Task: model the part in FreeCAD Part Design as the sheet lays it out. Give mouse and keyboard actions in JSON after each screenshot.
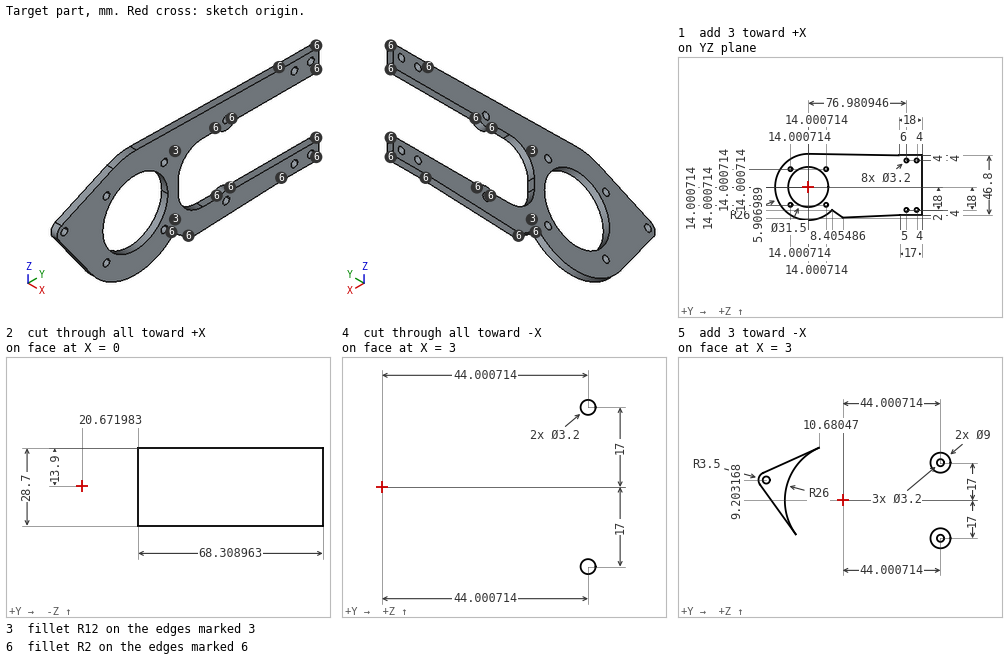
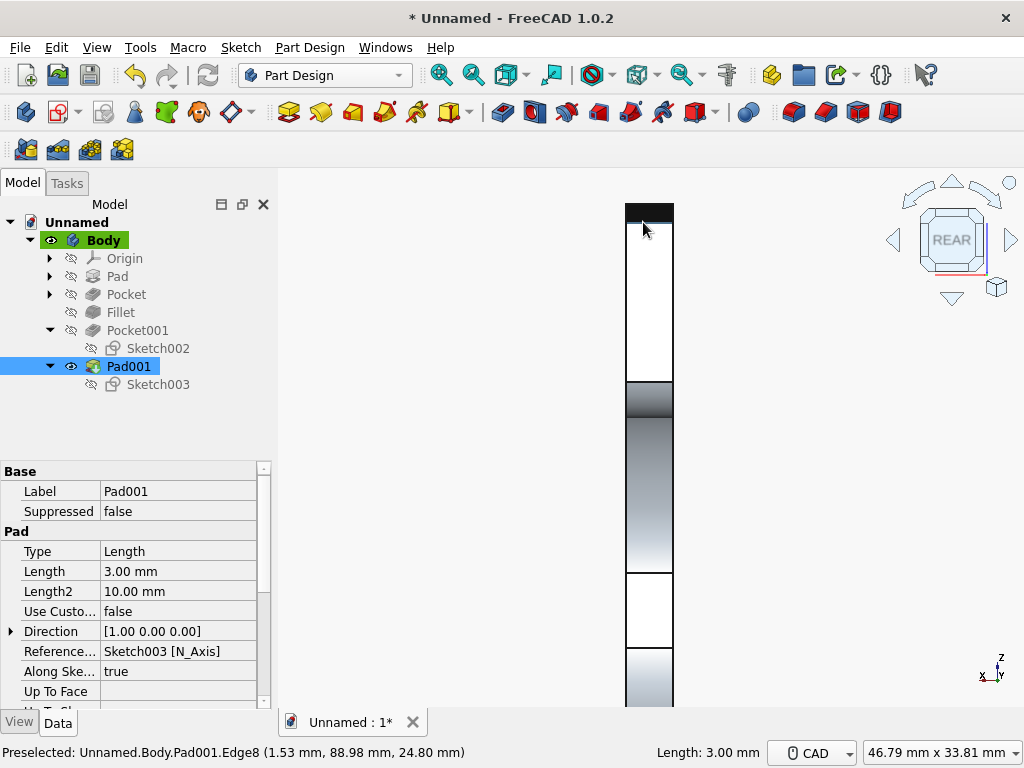
{"action": "left_click", "coordinate": [649, 381], "text": "ctrl"}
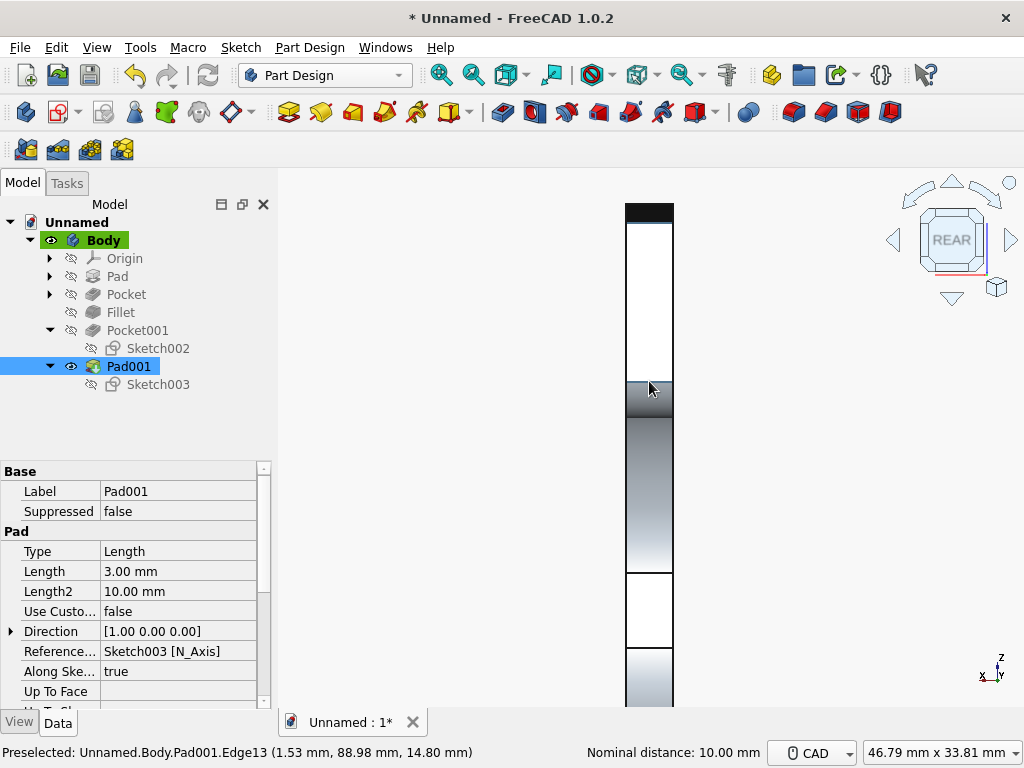
{"action": "left_click", "coordinate": [442, 76]}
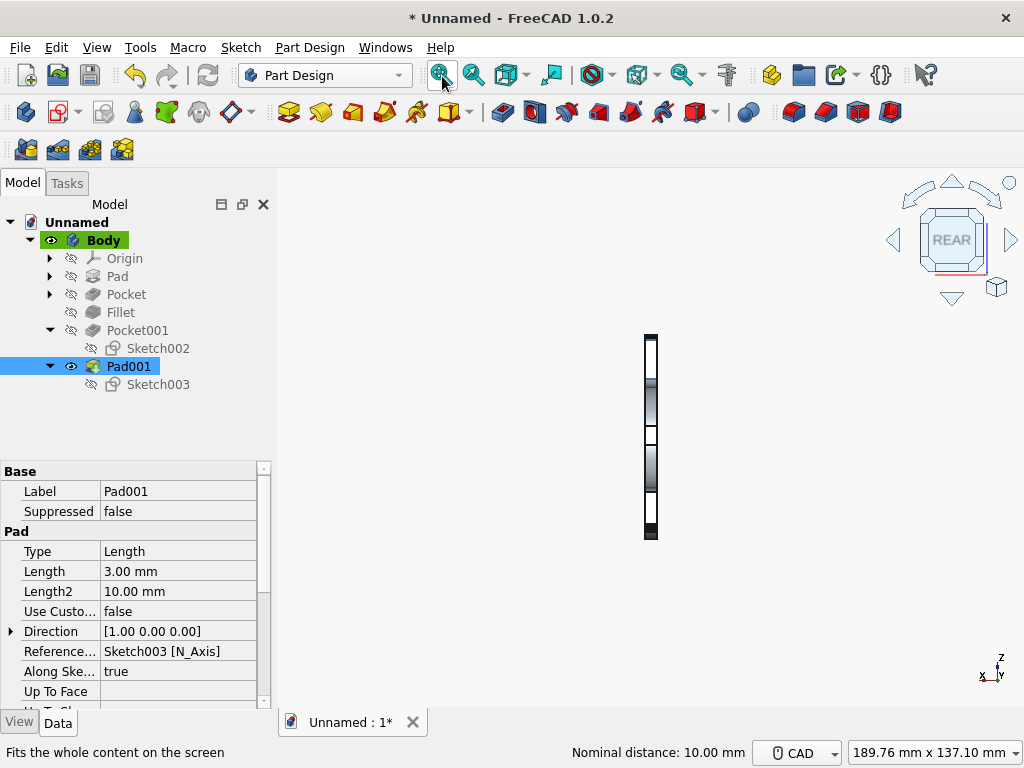
{"action": "key", "text": "6"}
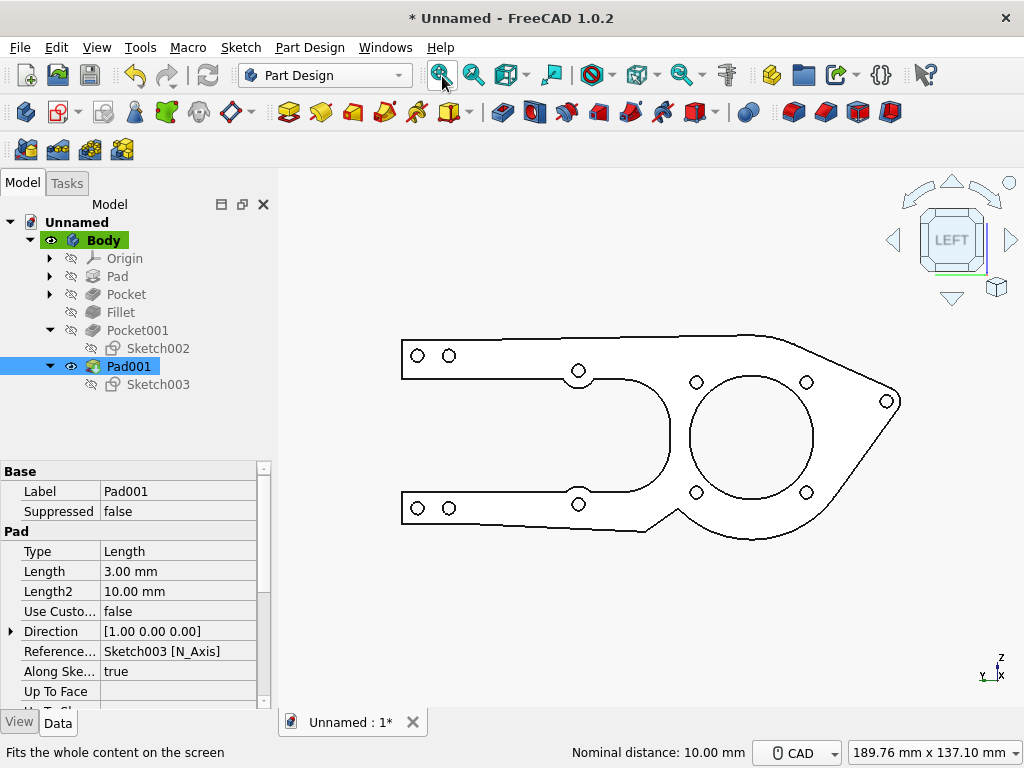
{"action": "scroll", "coordinate": [563, 378], "scroll_direction": "up", "scroll_amount": 7}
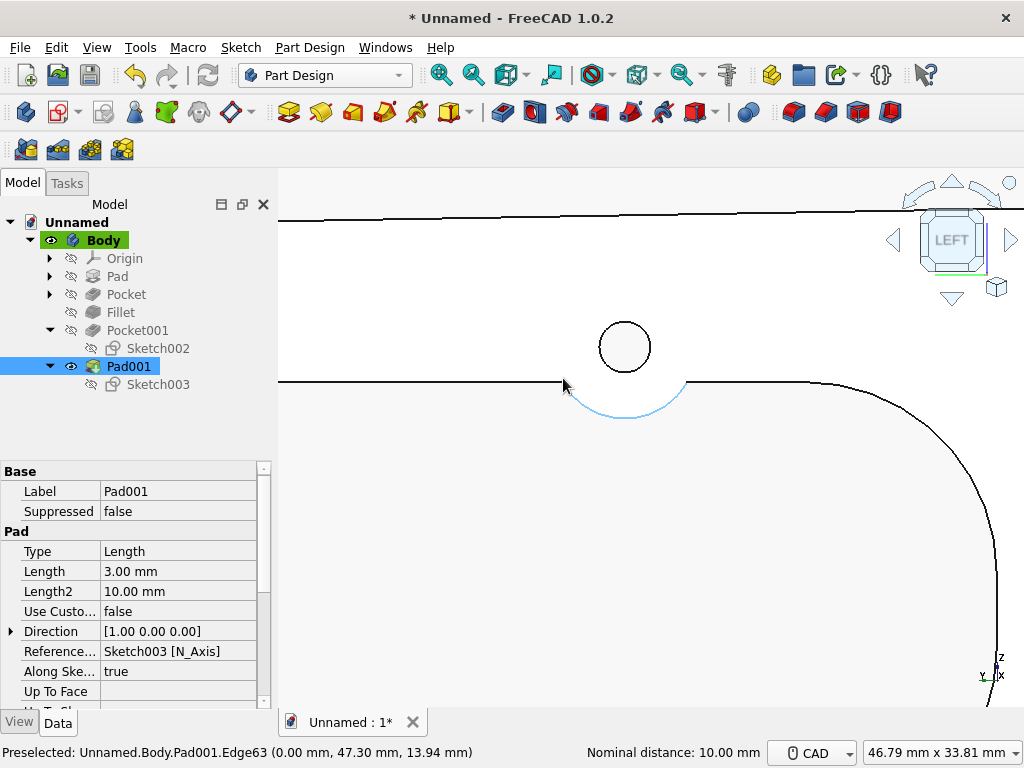
{"action": "left_click", "coordinate": [442, 76]}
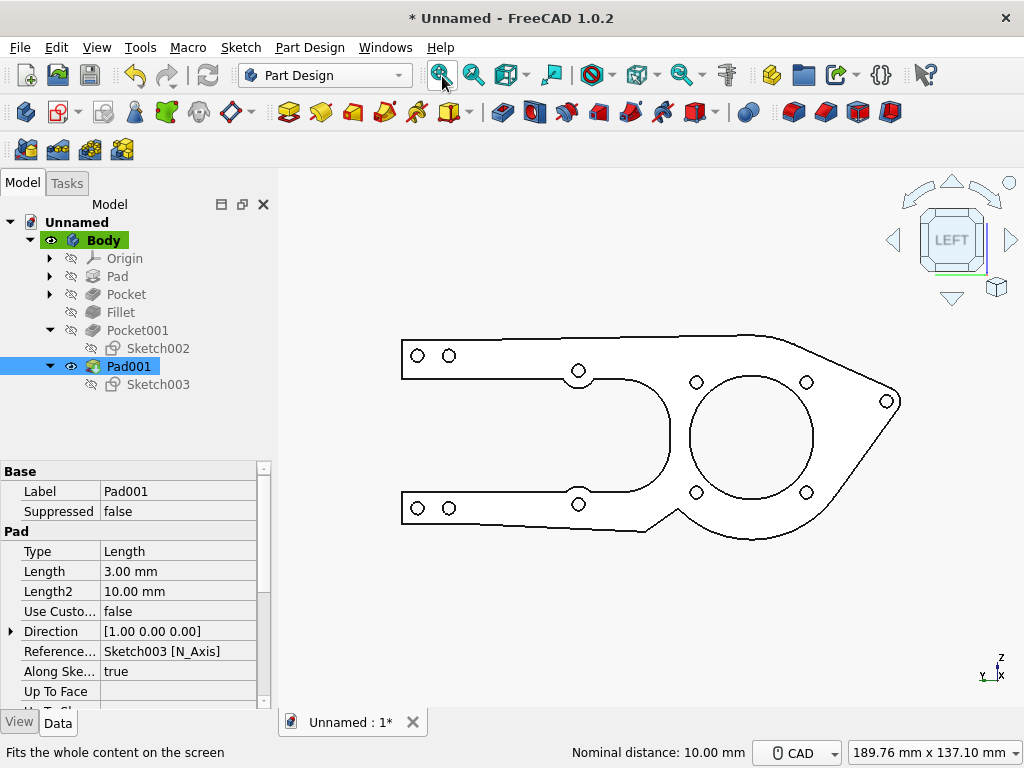
{"action": "key", "text": "v 3"}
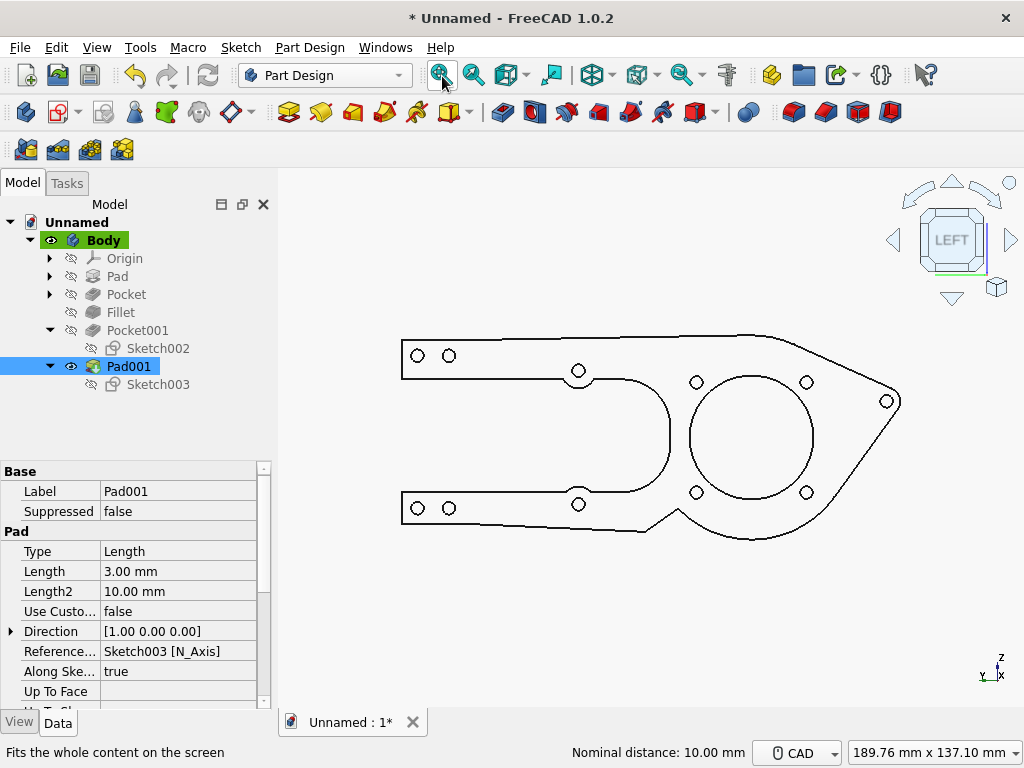
{"action": "key", "text": "0"}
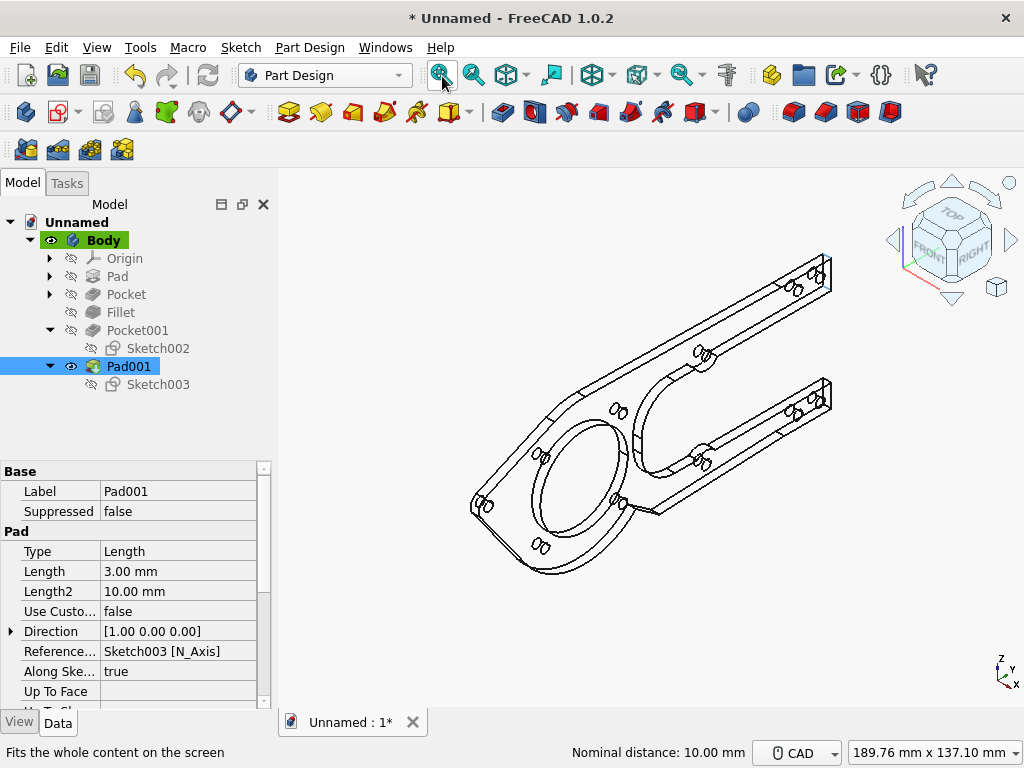
{"action": "left_click", "coordinate": [689, 364], "text": "ctrl"}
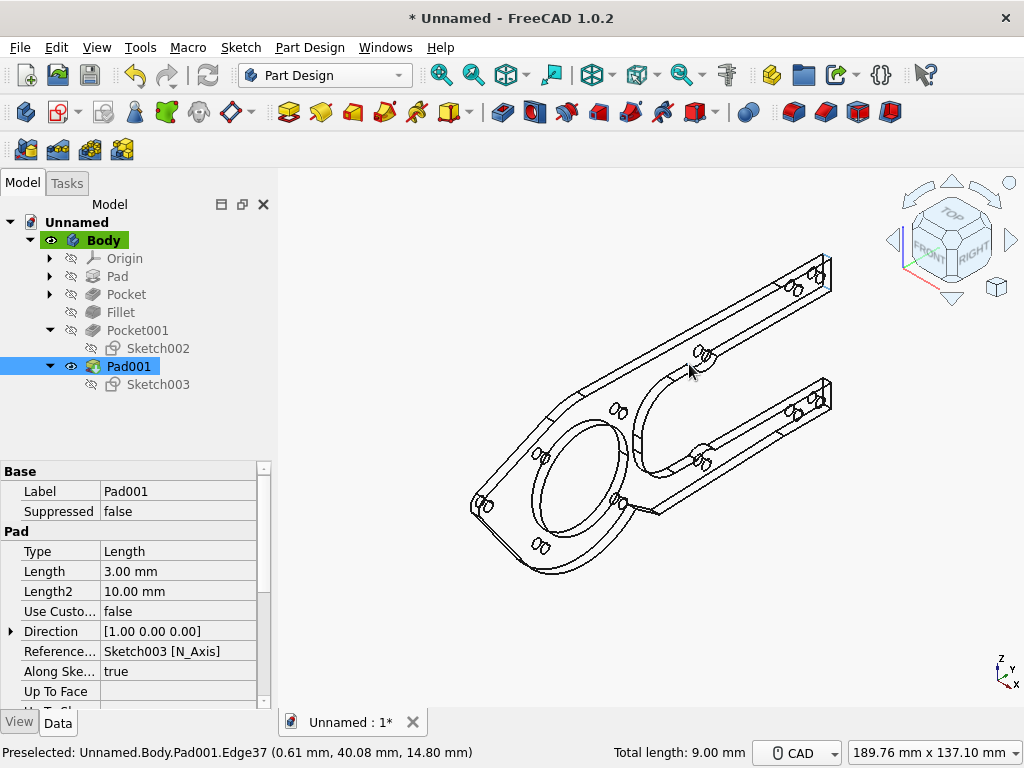
{"action": "left_click", "coordinate": [778, 431], "text": "ctrl"}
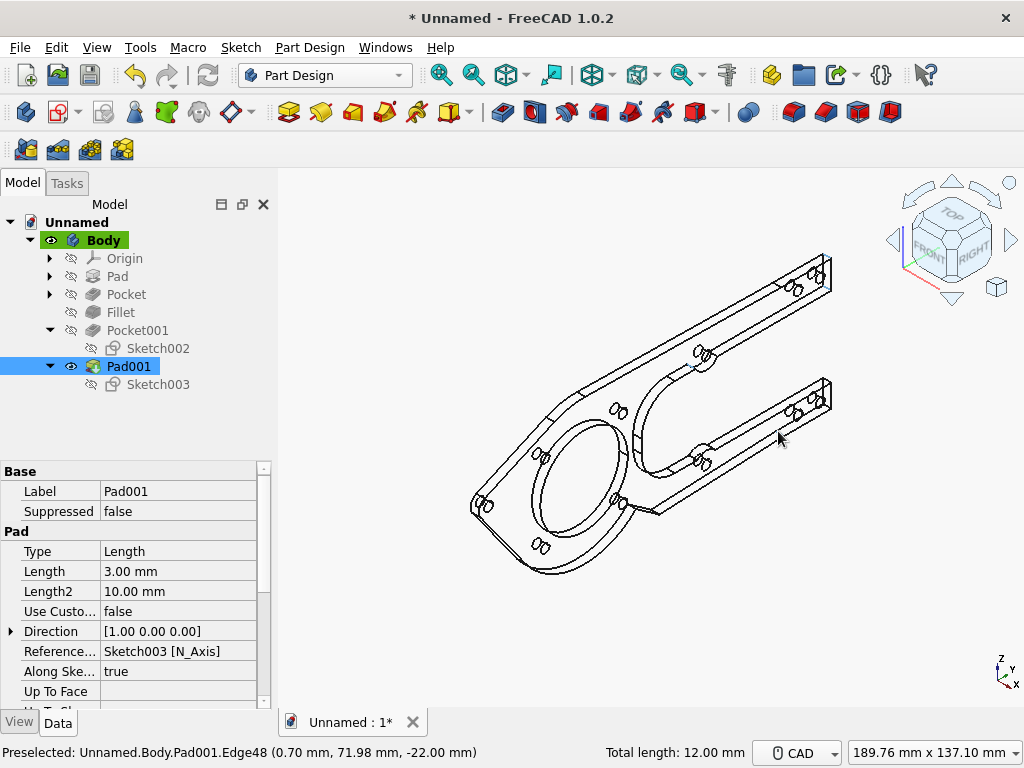
{"action": "left_click", "coordinate": [691, 455], "text": "ctrl"}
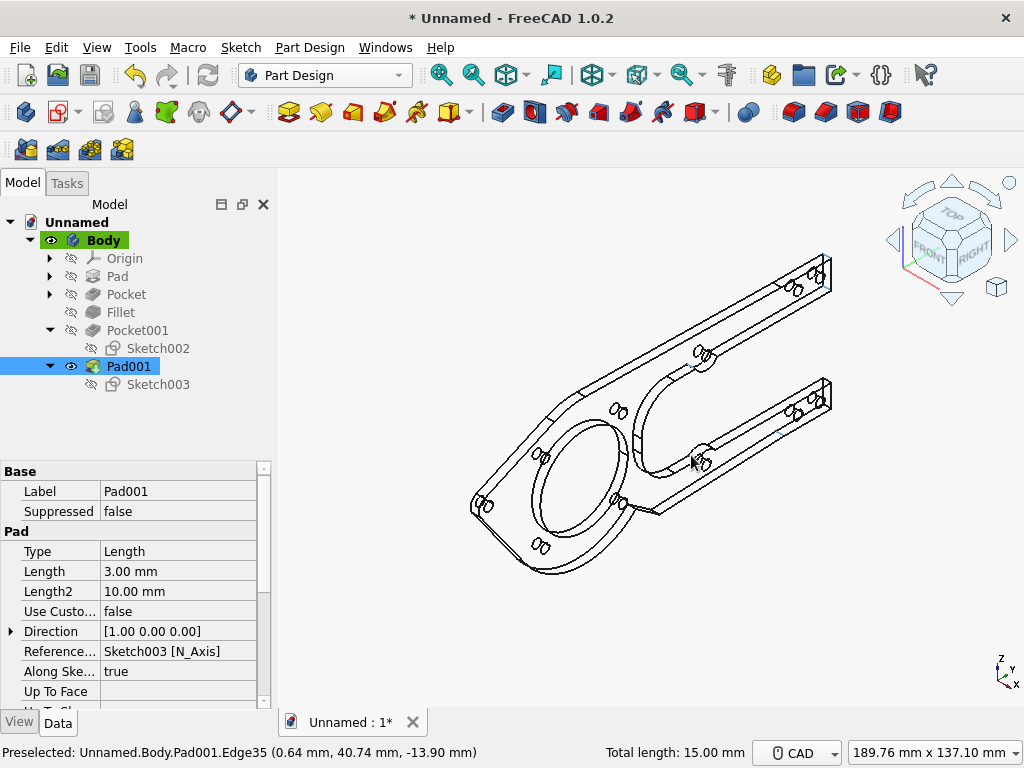
{"action": "left_click", "coordinate": [825, 378], "text": "ctrl"}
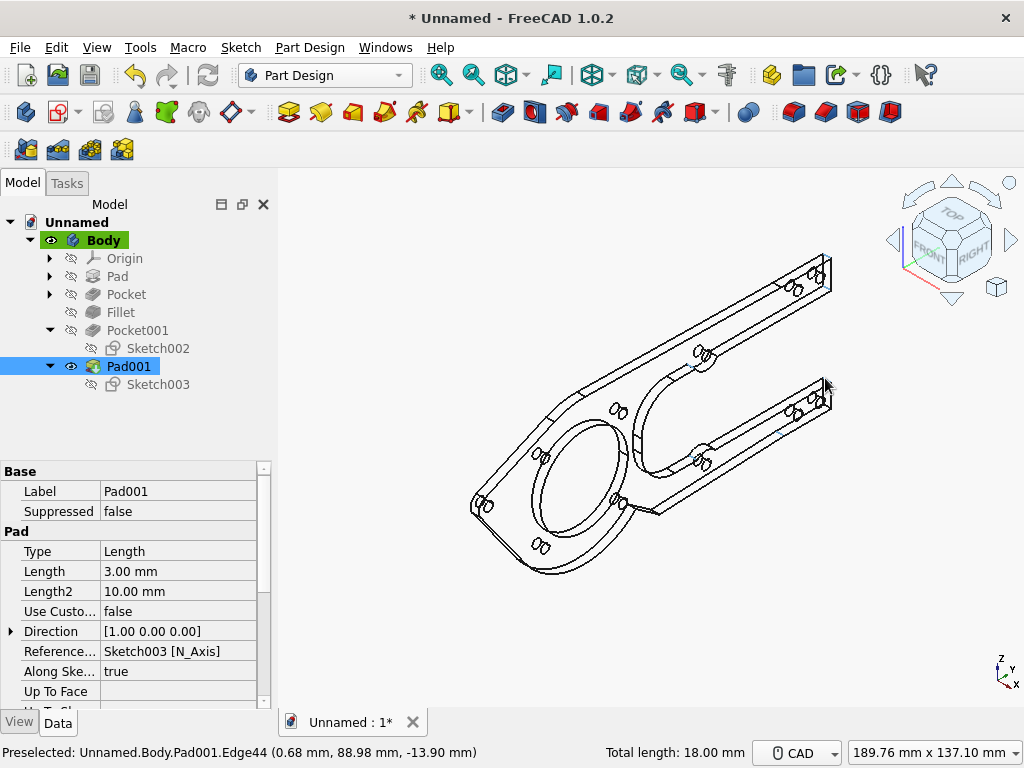
{"action": "scroll", "coordinate": [713, 353], "scroll_direction": "up", "scroll_amount": 7}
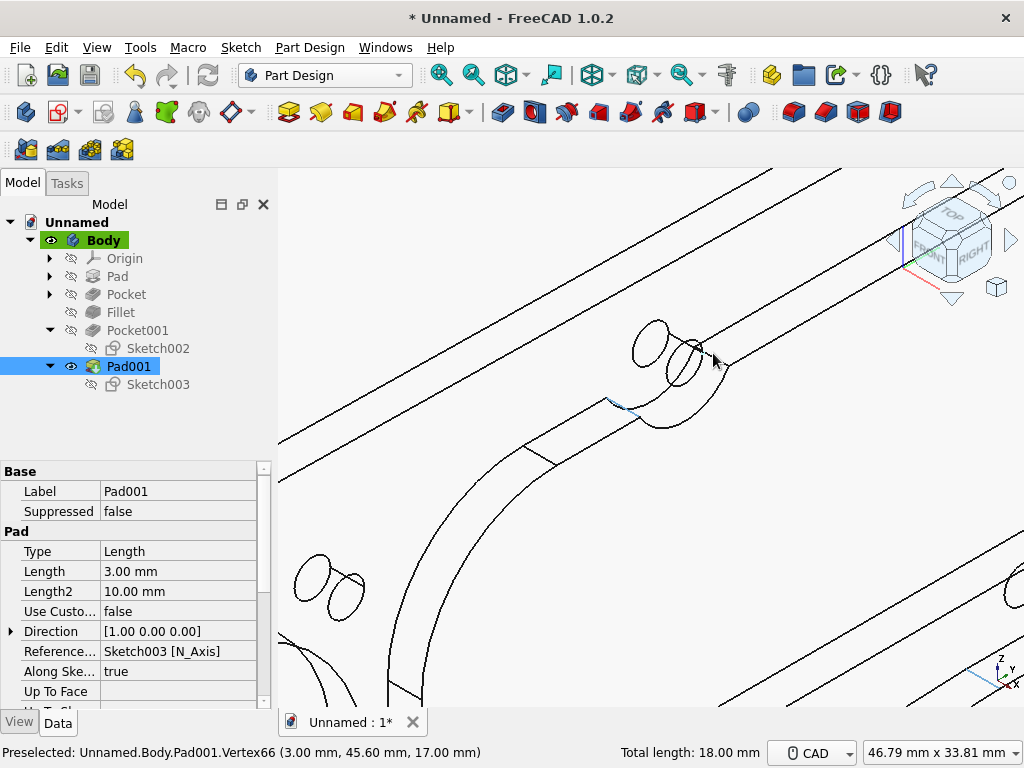
{"action": "left_click", "coordinate": [712, 355], "text": "ctrl"}